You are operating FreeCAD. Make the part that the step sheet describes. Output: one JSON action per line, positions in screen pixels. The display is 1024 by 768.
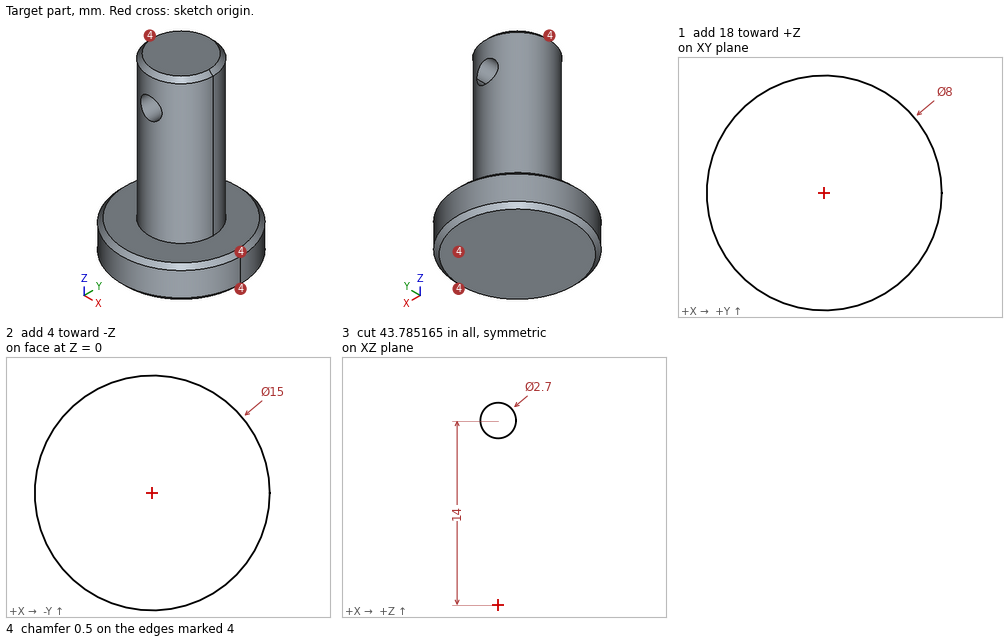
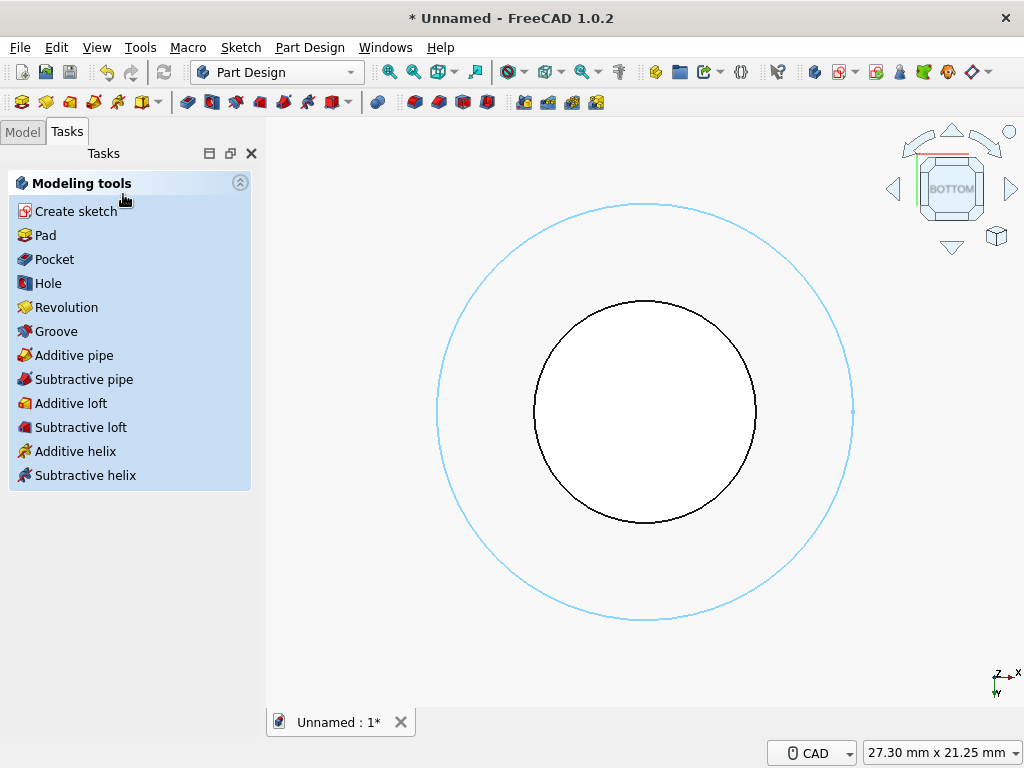
{"action": "left_click", "coordinate": [22, 102]}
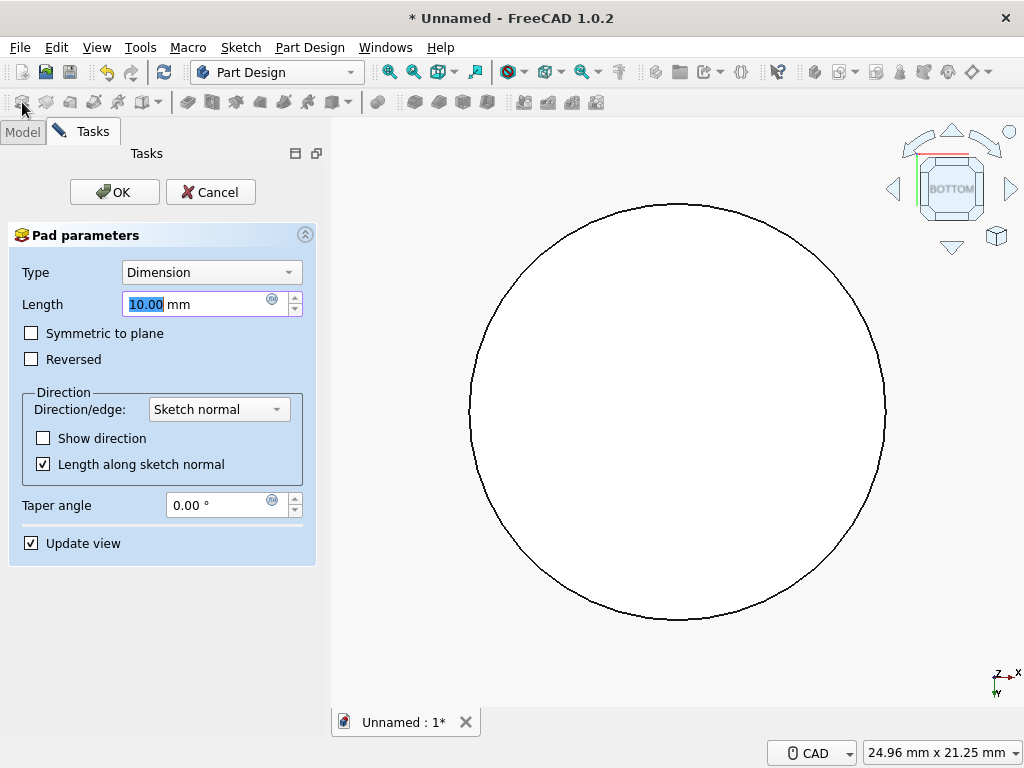
{"action": "type", "text": "4"}
{"action": "key", "text": "Tab"}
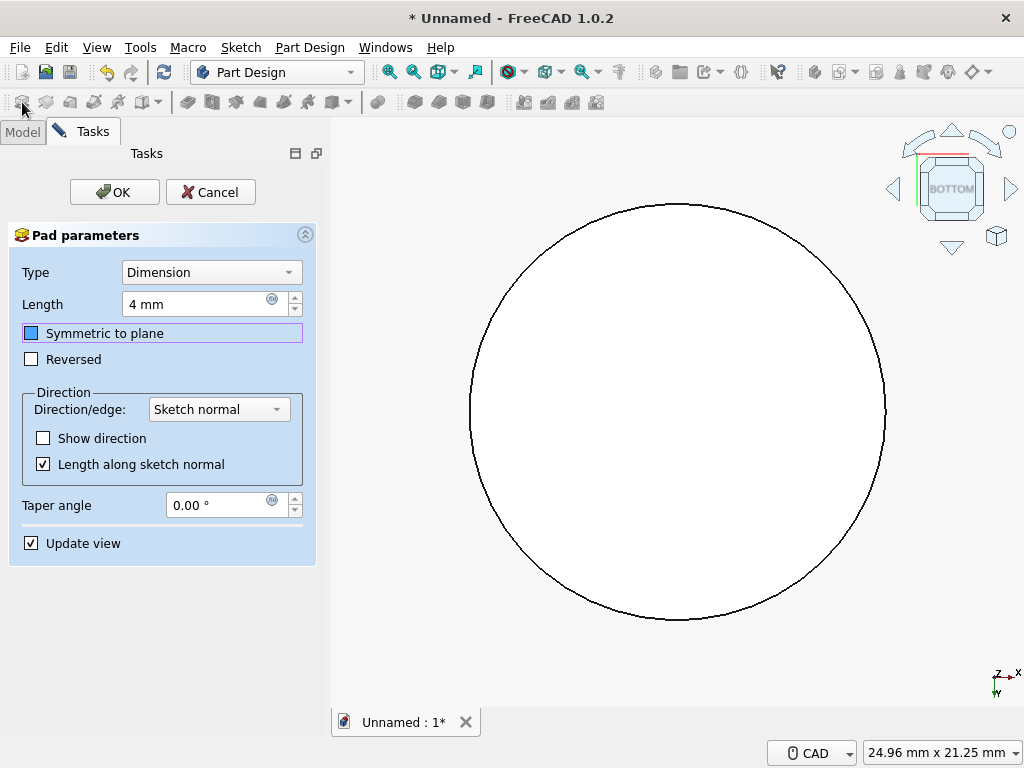
{"action": "left_click", "coordinate": [115, 192]}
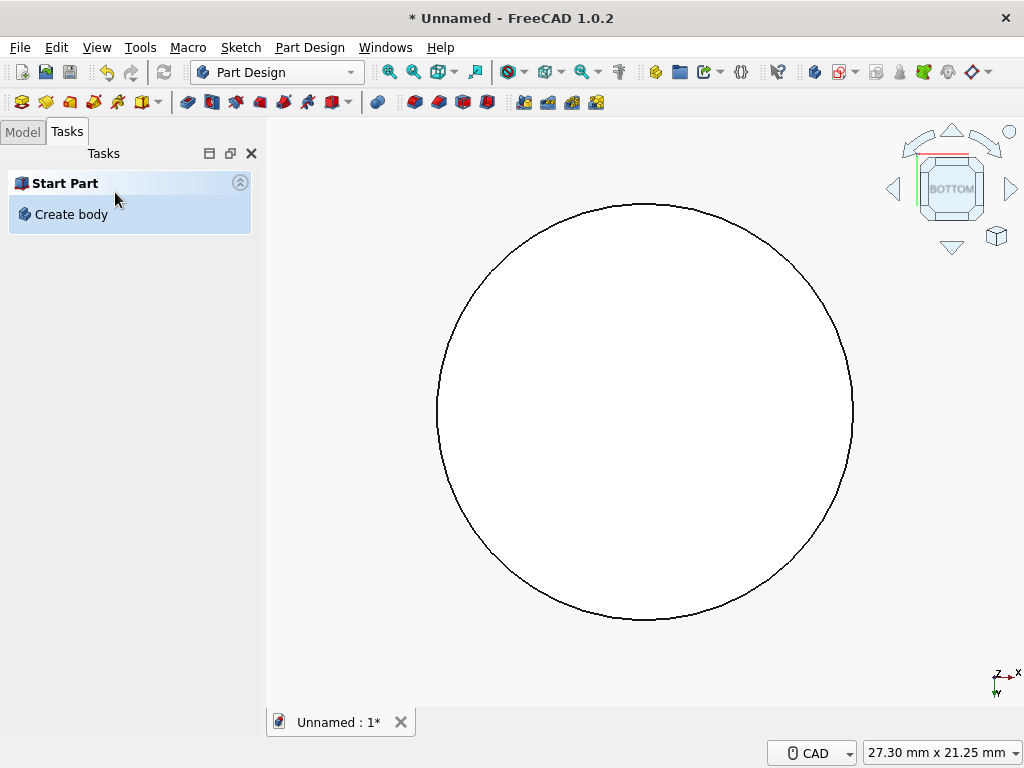
{"action": "left_click", "coordinate": [840, 72]}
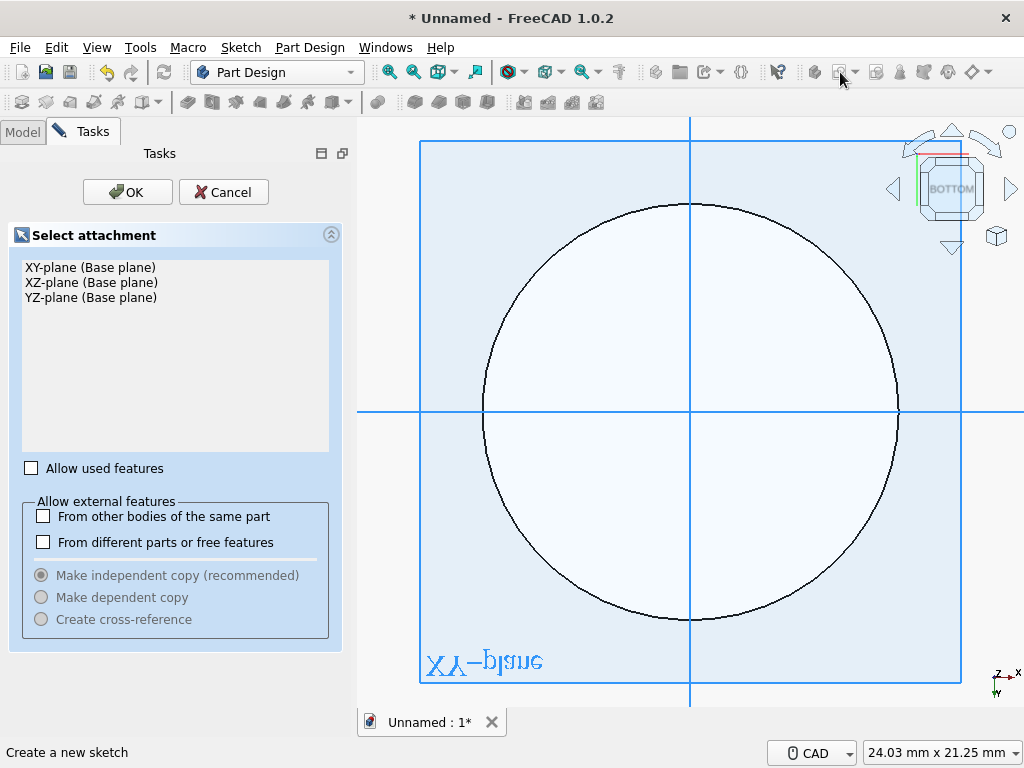
{"action": "left_click", "coordinate": [82, 282]}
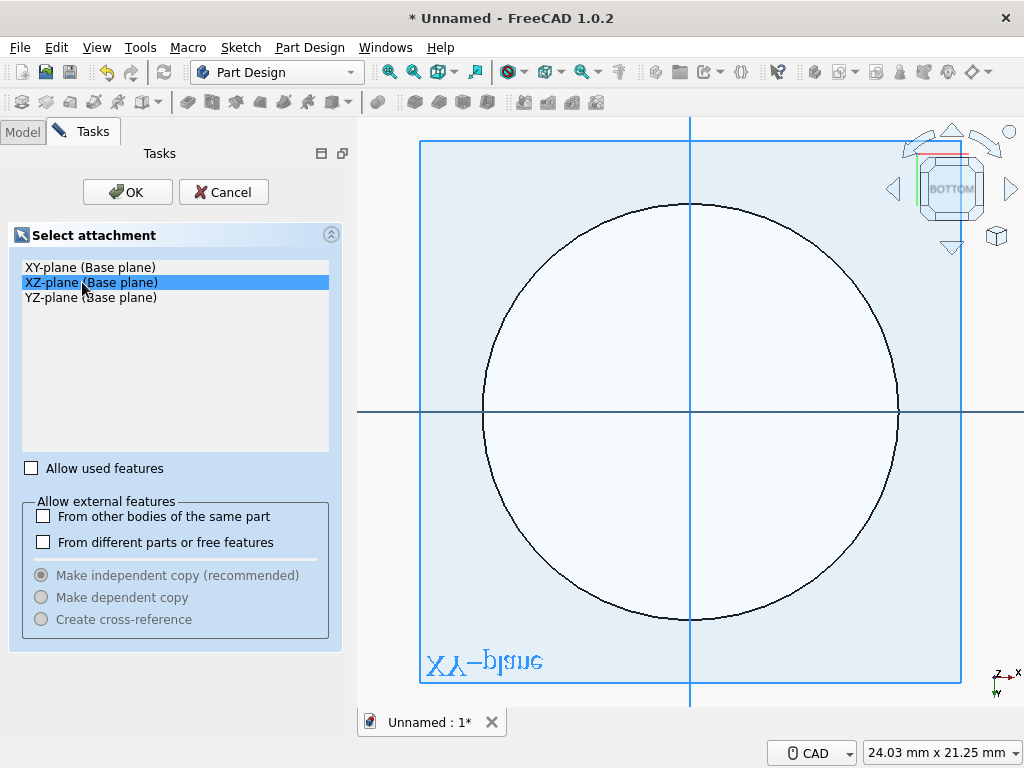
{"action": "left_click", "coordinate": [128, 192]}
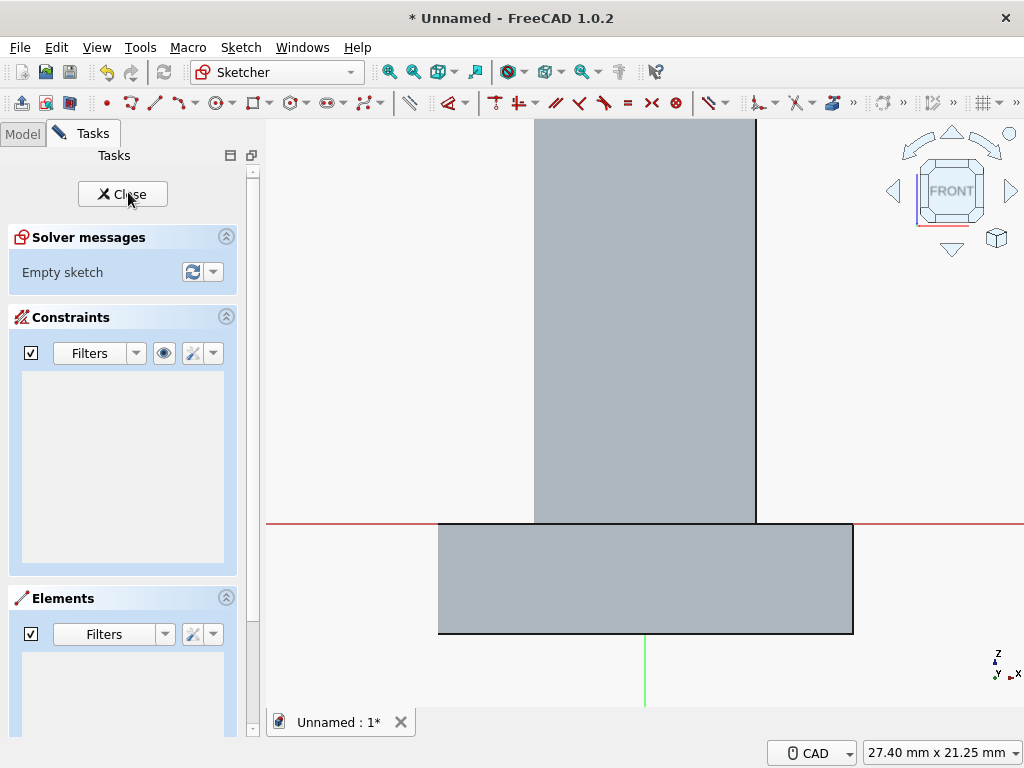
{"action": "left_click", "coordinate": [70, 104]}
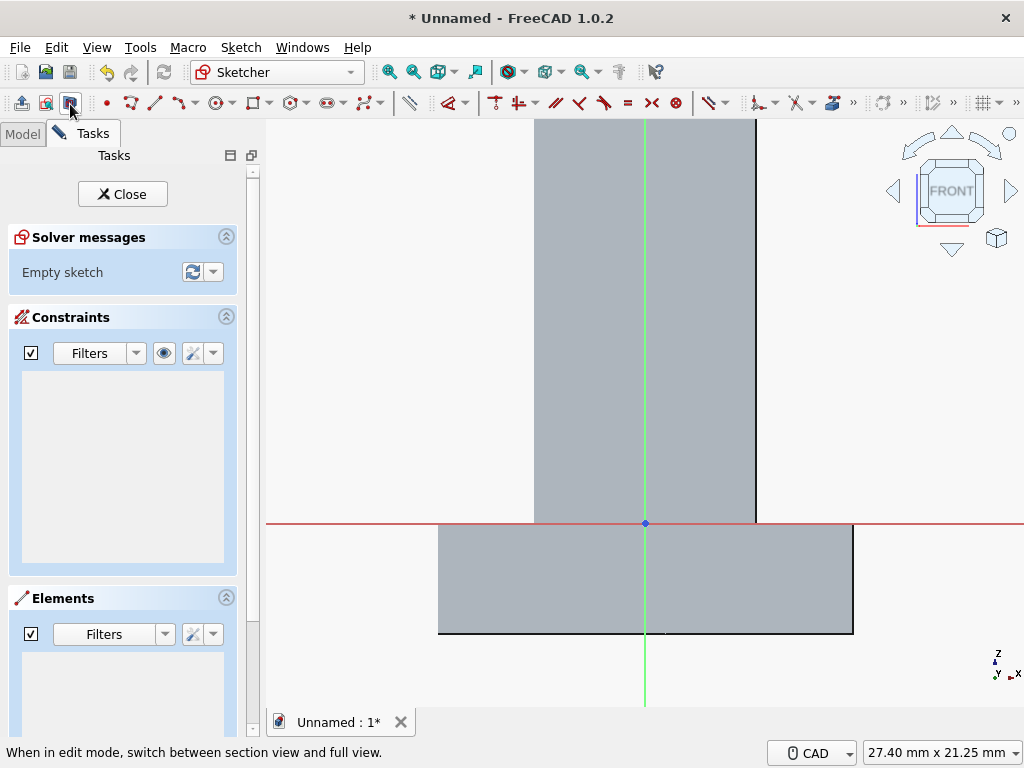
{"action": "scroll", "coordinate": [576, 413], "scroll_direction": "down", "scroll_amount": 5}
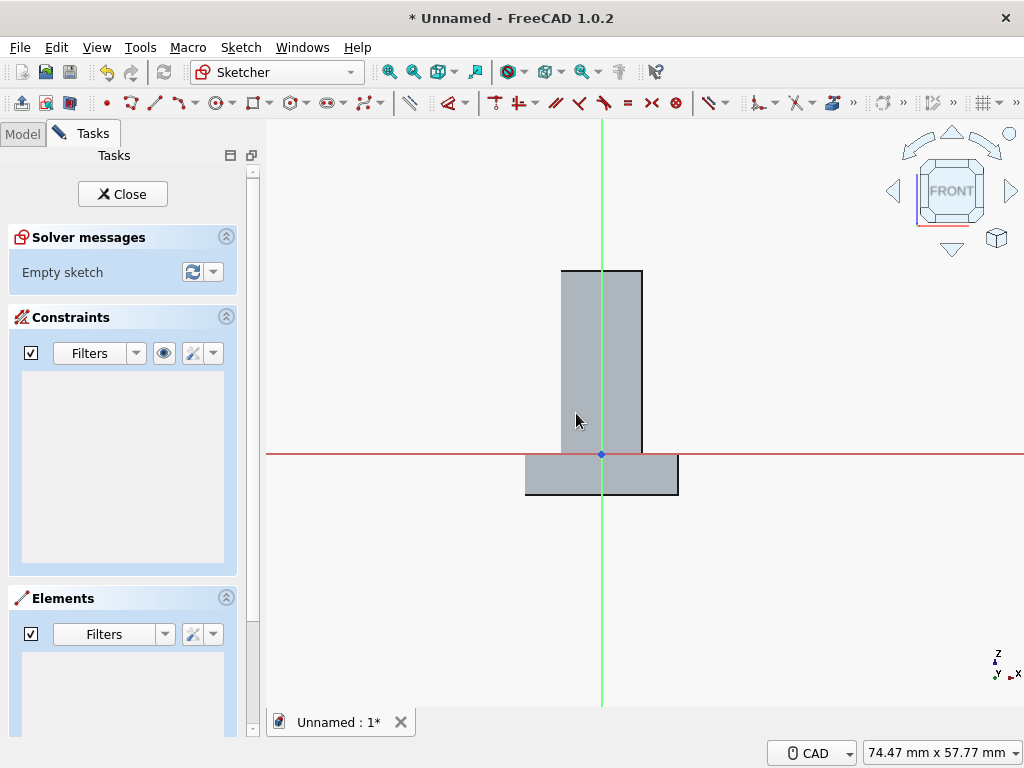
{"action": "scroll", "coordinate": [604, 303], "scroll_direction": "up", "scroll_amount": 13}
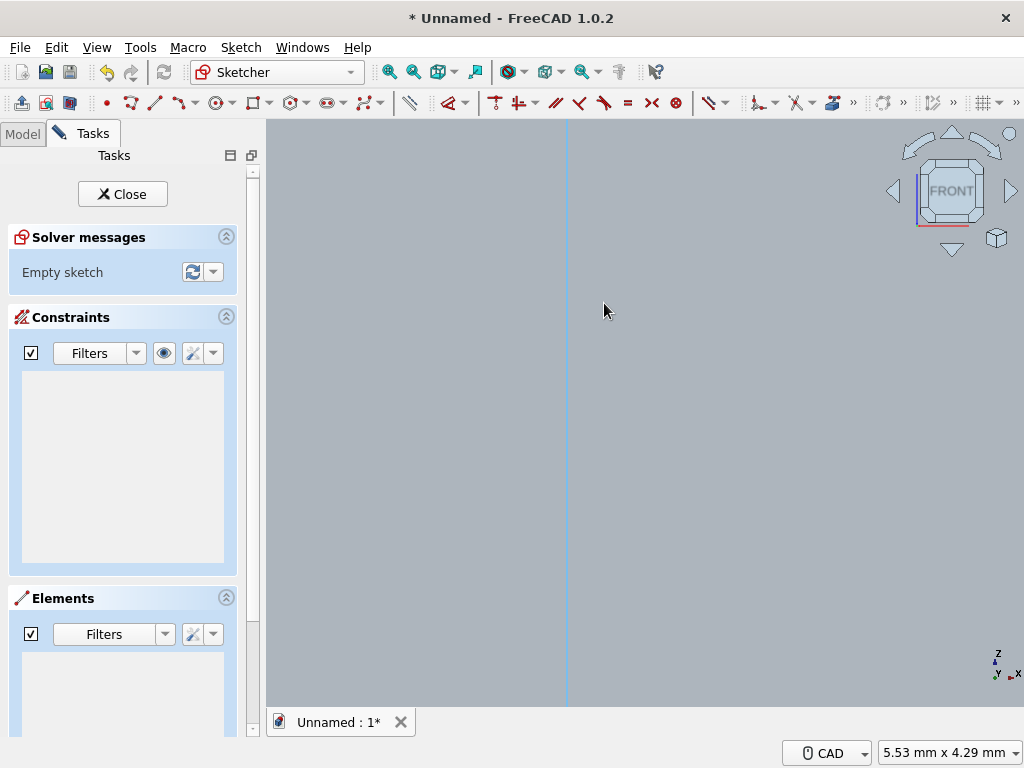
{"action": "left_click", "coordinate": [216, 104]}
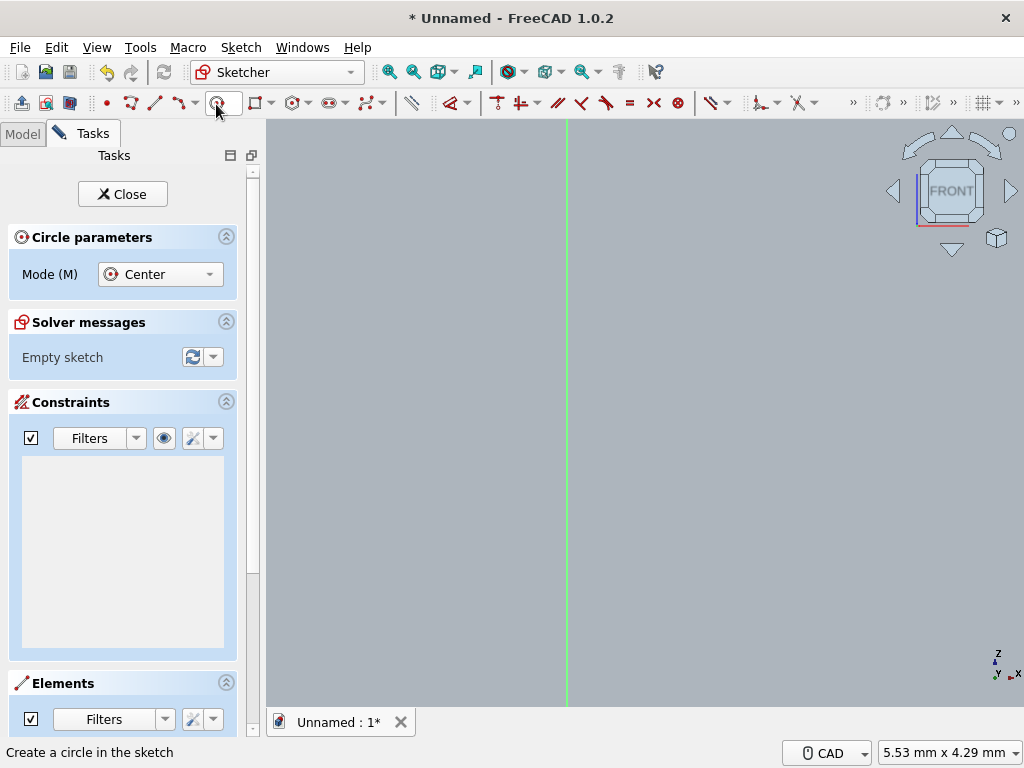
{"action": "left_click", "coordinate": [567, 414]}
{"action": "left_click", "coordinate": [698, 283]}
{"action": "key", "text": "Escape"}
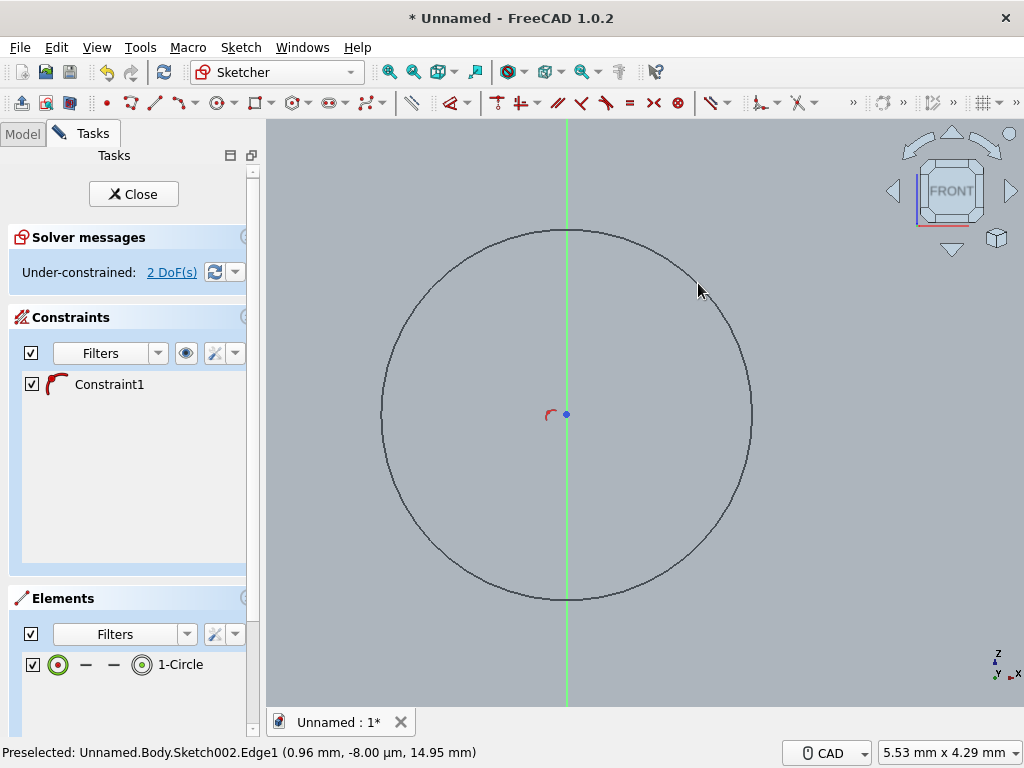
{"action": "left_click", "coordinate": [450, 104]}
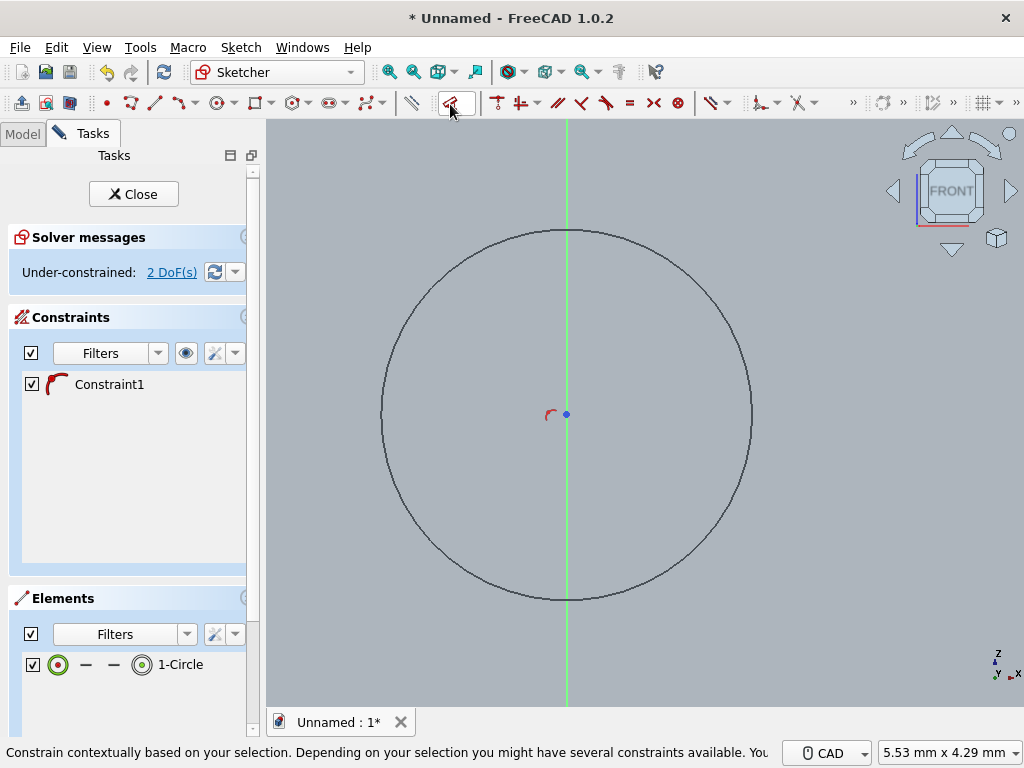
{"action": "left_click", "coordinate": [697, 283]}
{"action": "left_click", "coordinate": [719, 260]}